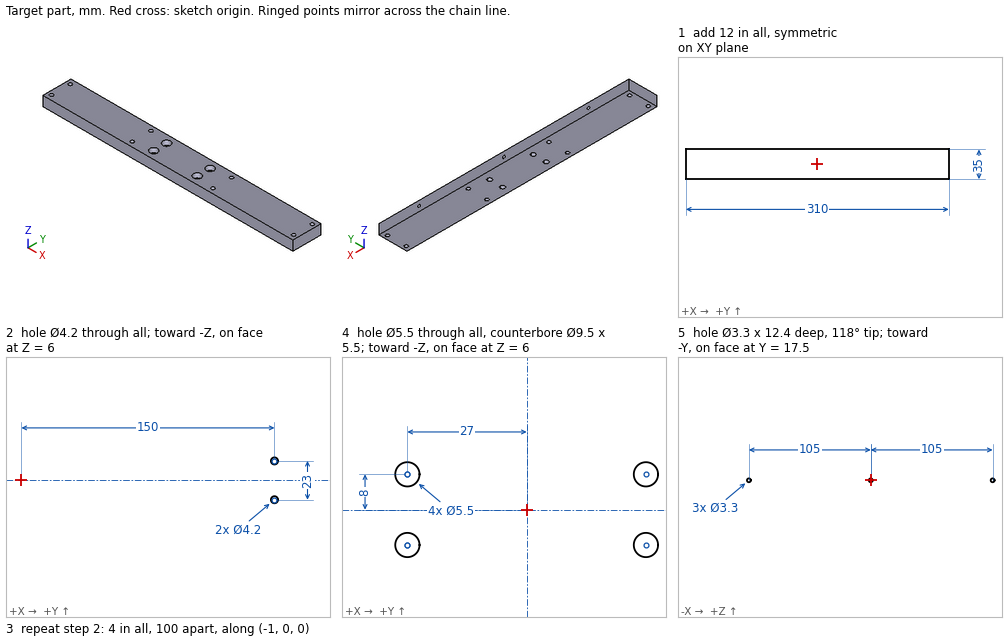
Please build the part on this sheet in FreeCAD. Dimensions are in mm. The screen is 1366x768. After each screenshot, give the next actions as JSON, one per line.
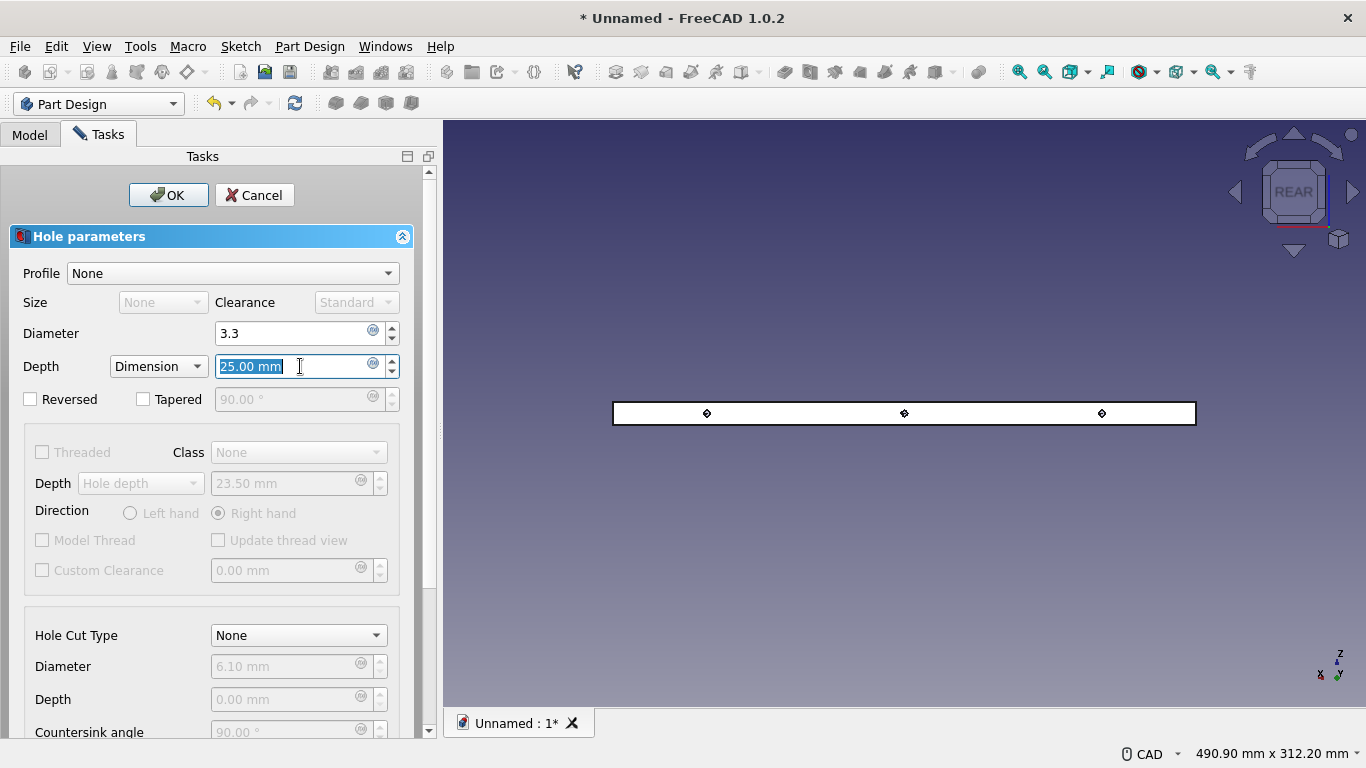
{"action": "type", "text": "12.4"}
{"action": "key", "text": "Tab"}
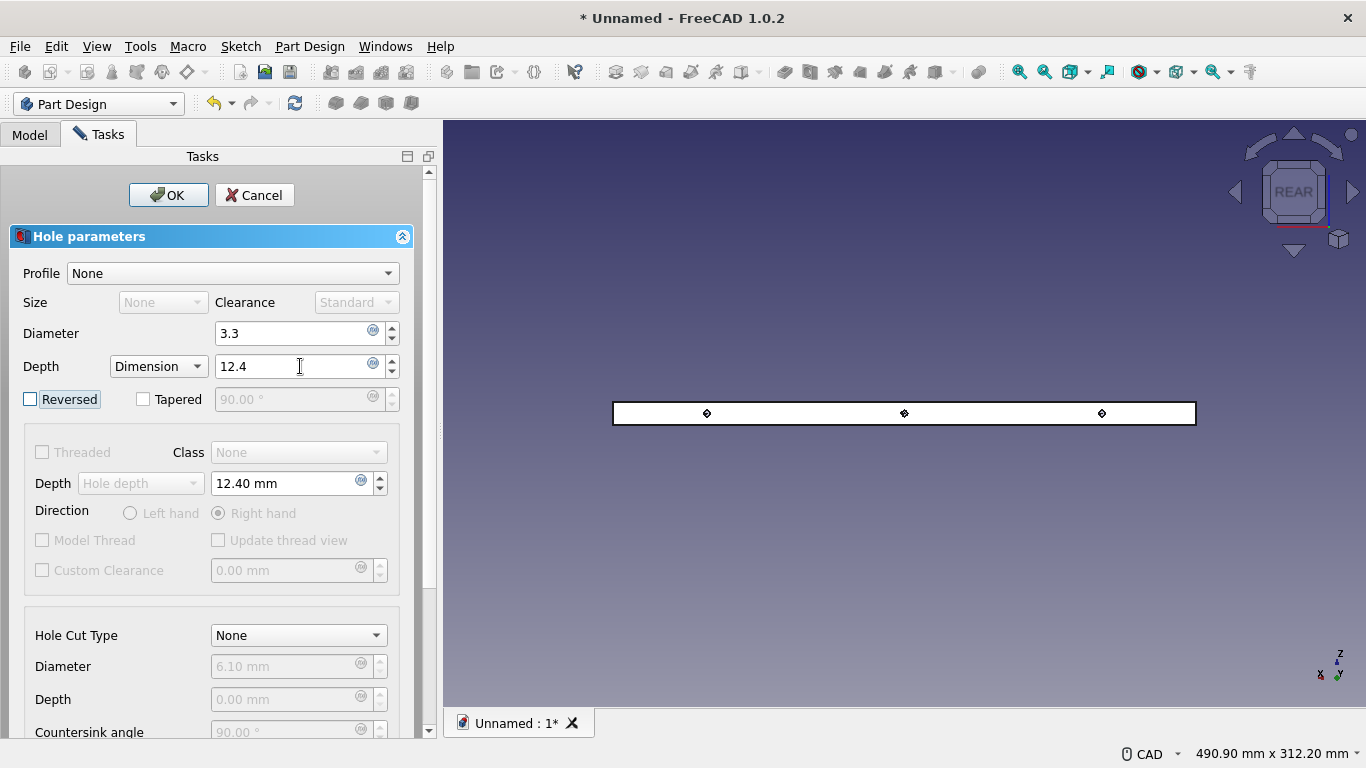
{"action": "left_click", "coordinate": [169, 195]}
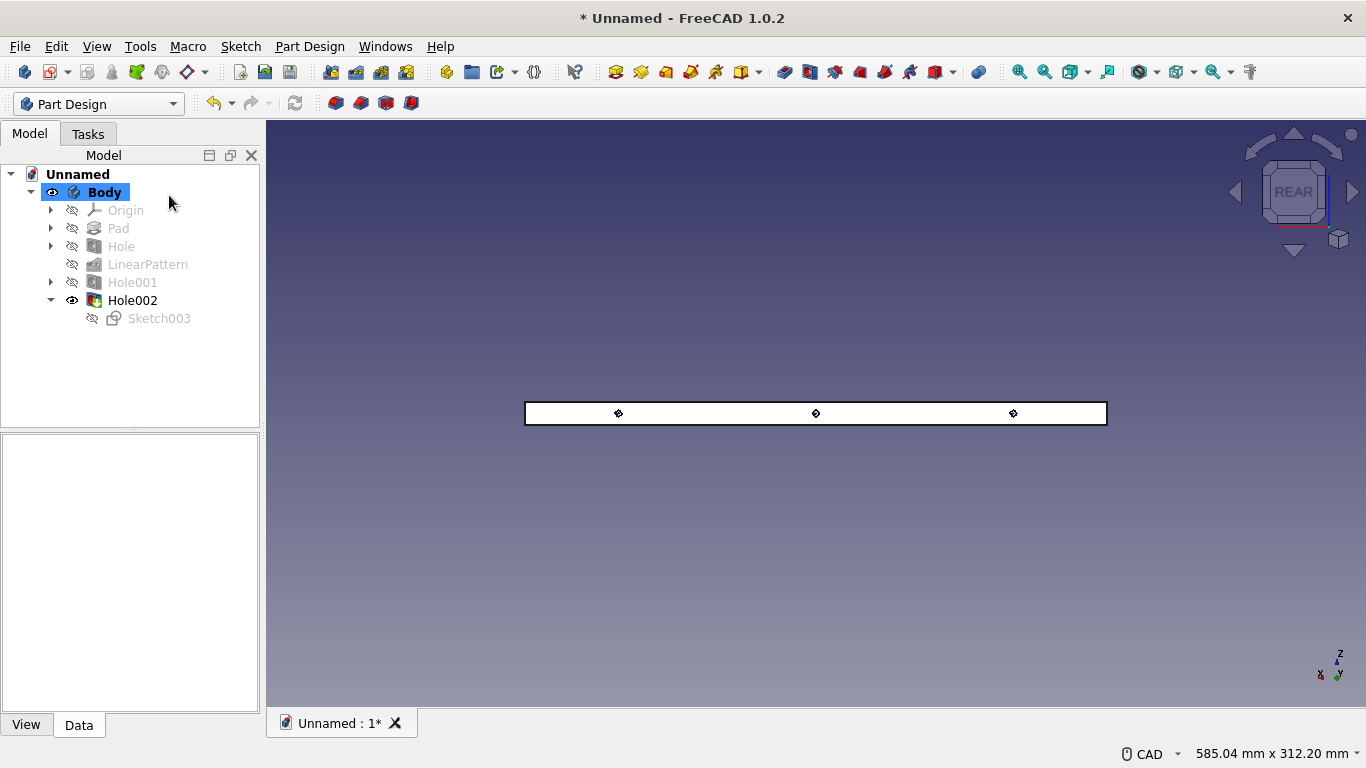
{"action": "key", "text": "0"}